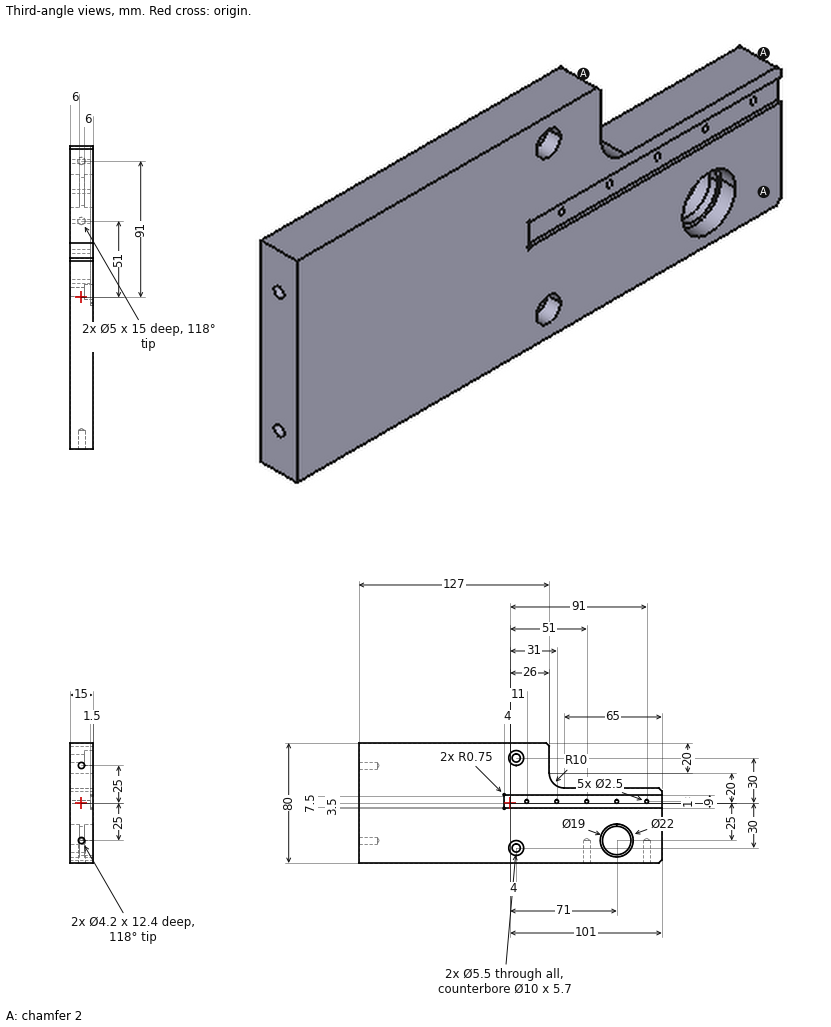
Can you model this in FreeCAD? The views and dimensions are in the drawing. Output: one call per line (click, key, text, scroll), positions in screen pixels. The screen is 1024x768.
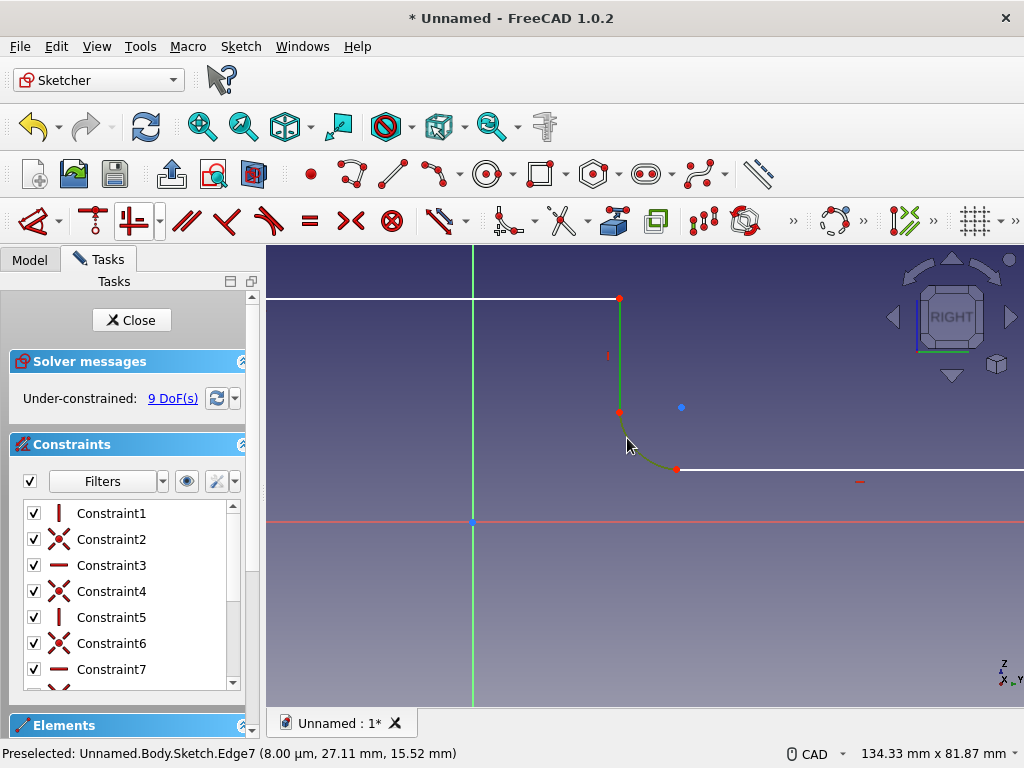
click(269, 222)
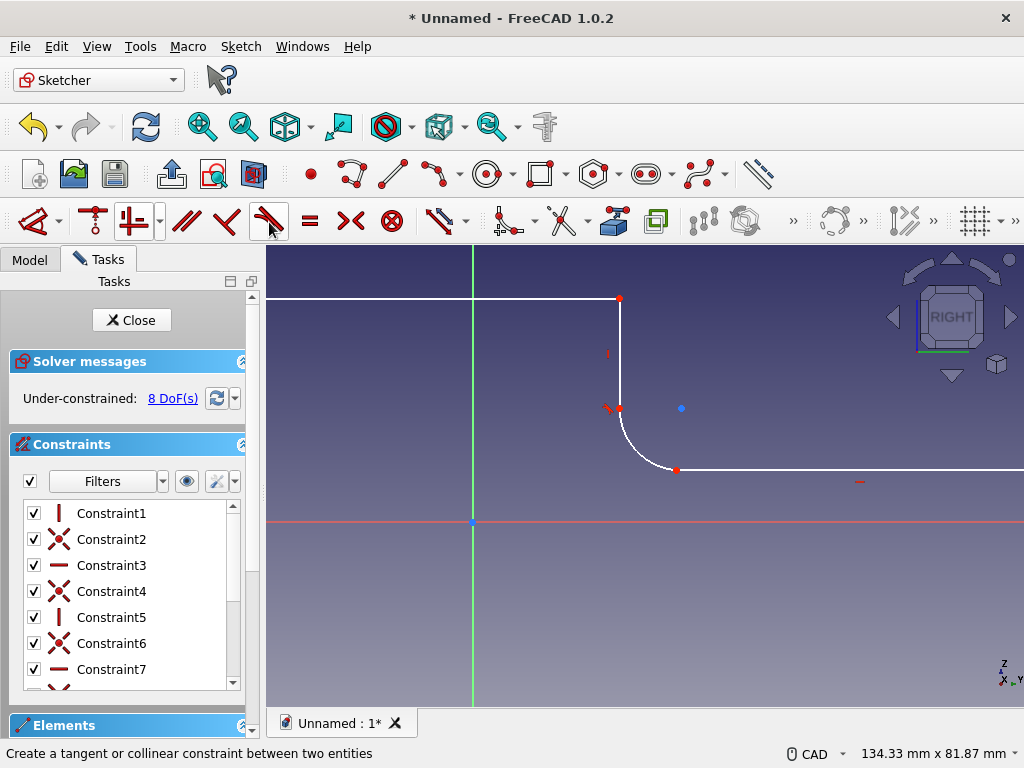
click(787, 470)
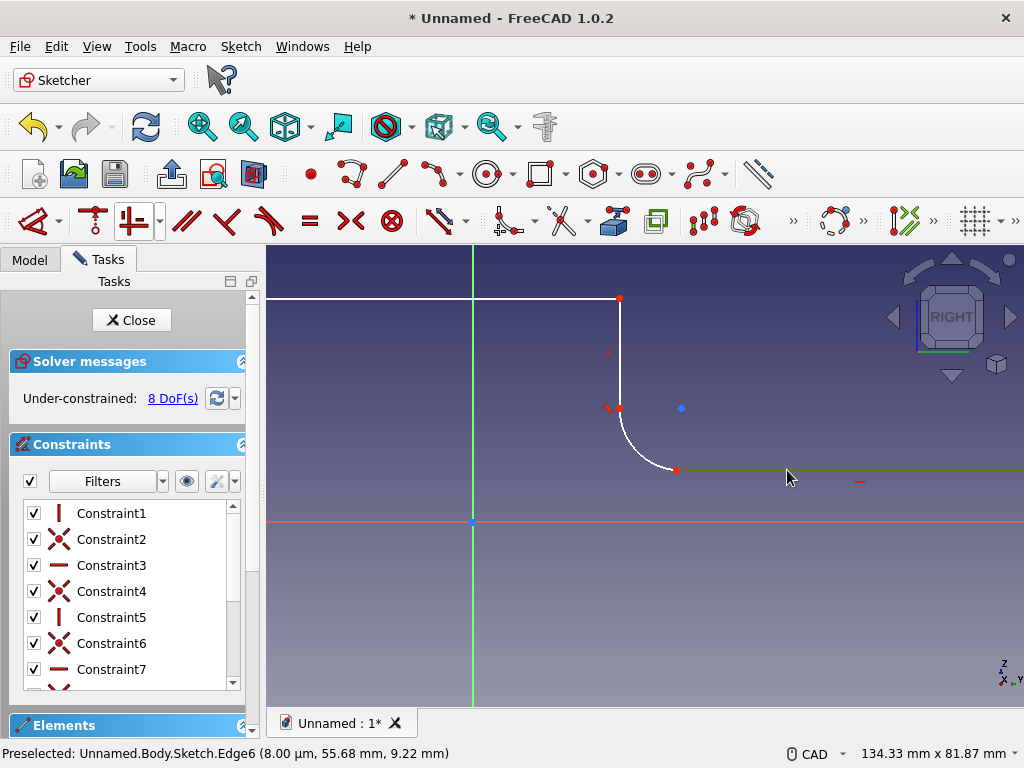
click(626, 435)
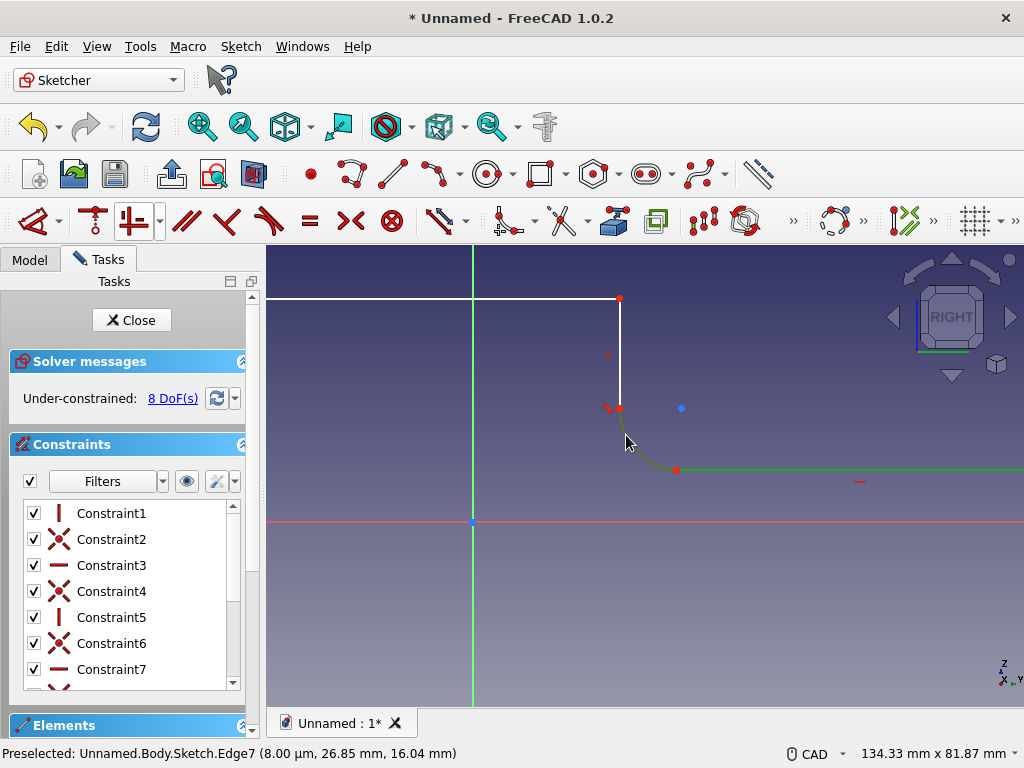
click(269, 222)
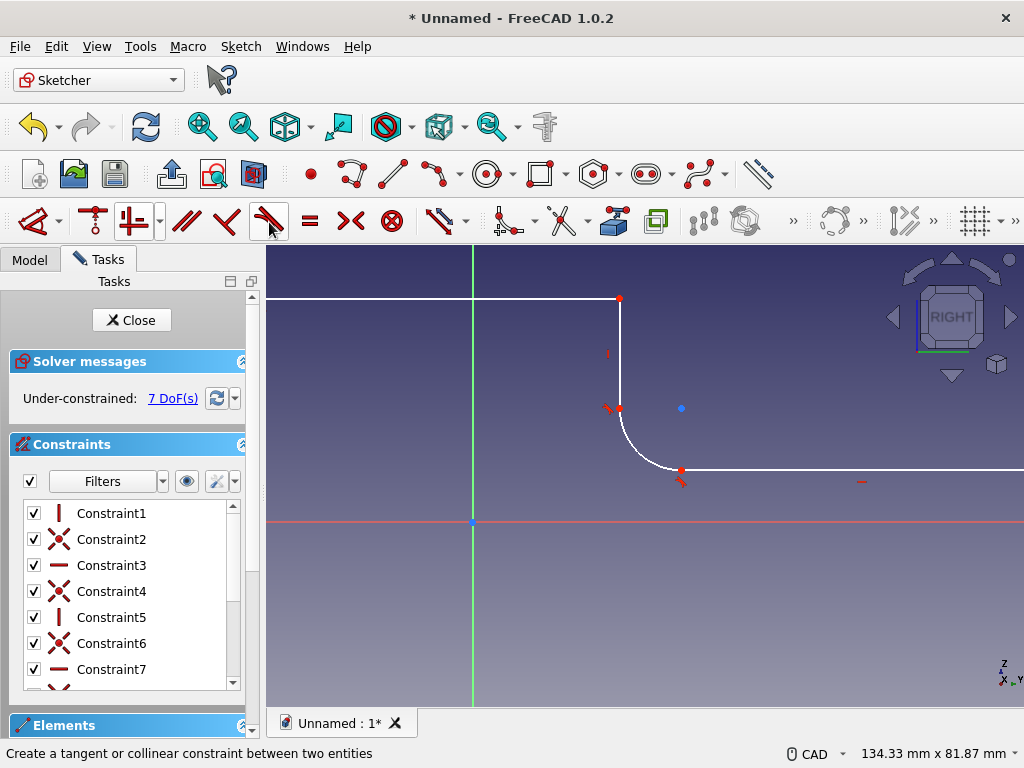
click(32, 222)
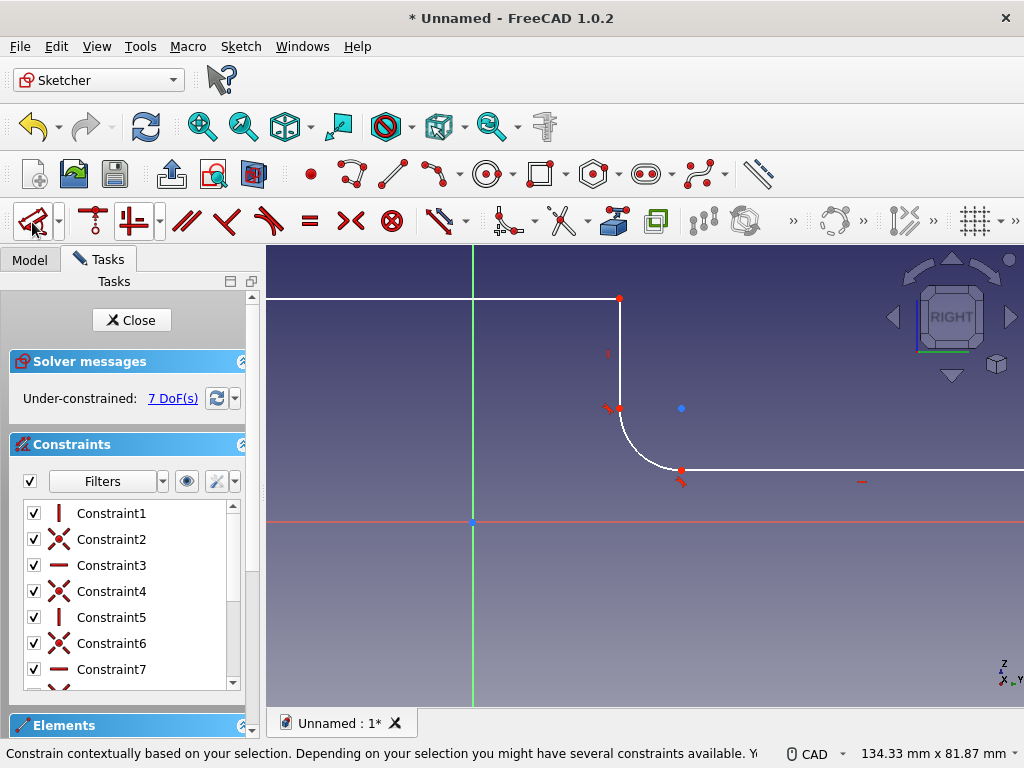
click(627, 437)
click(599, 452)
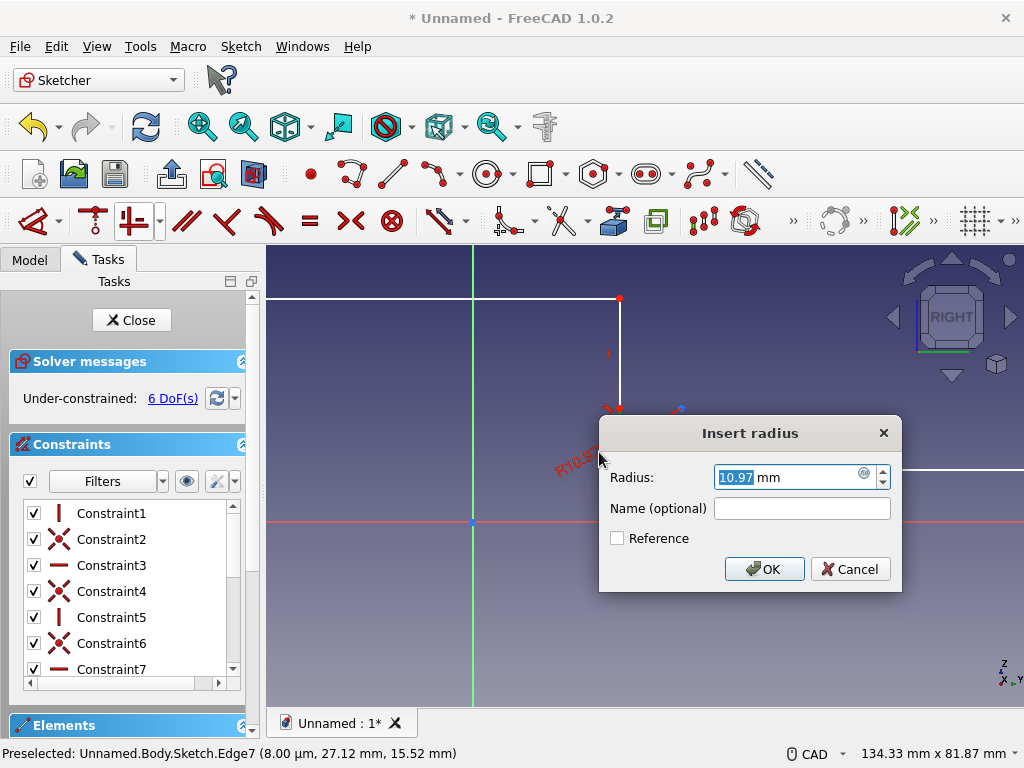
text(10)
key(Return)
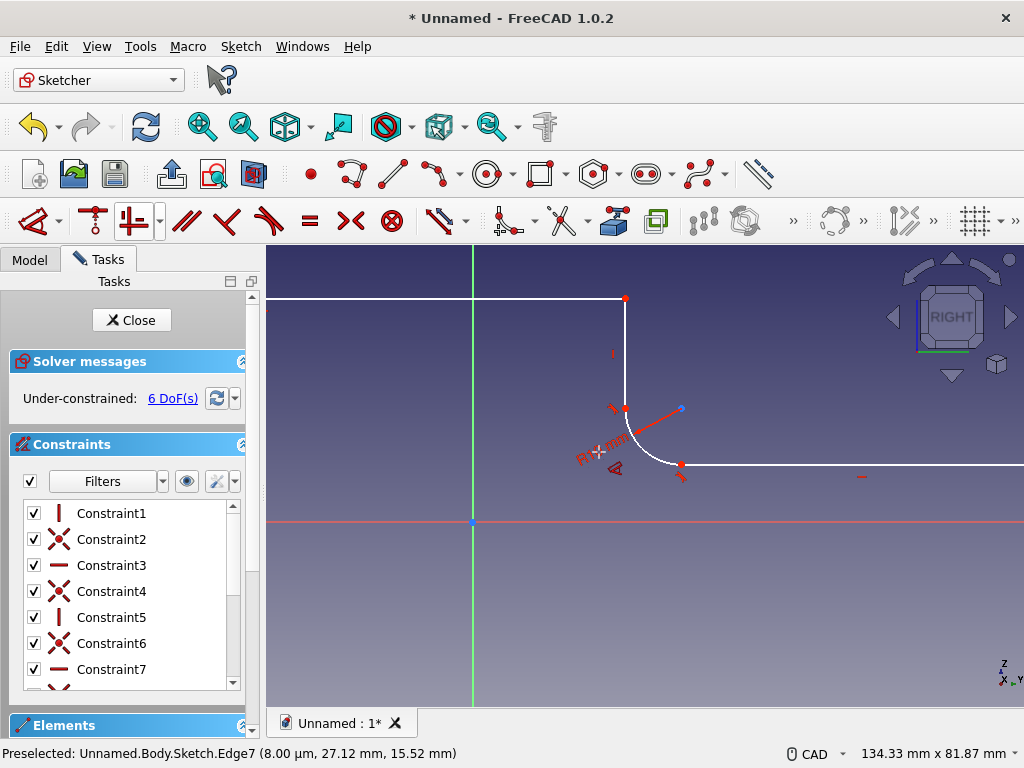
click(625, 376)
click(659, 354)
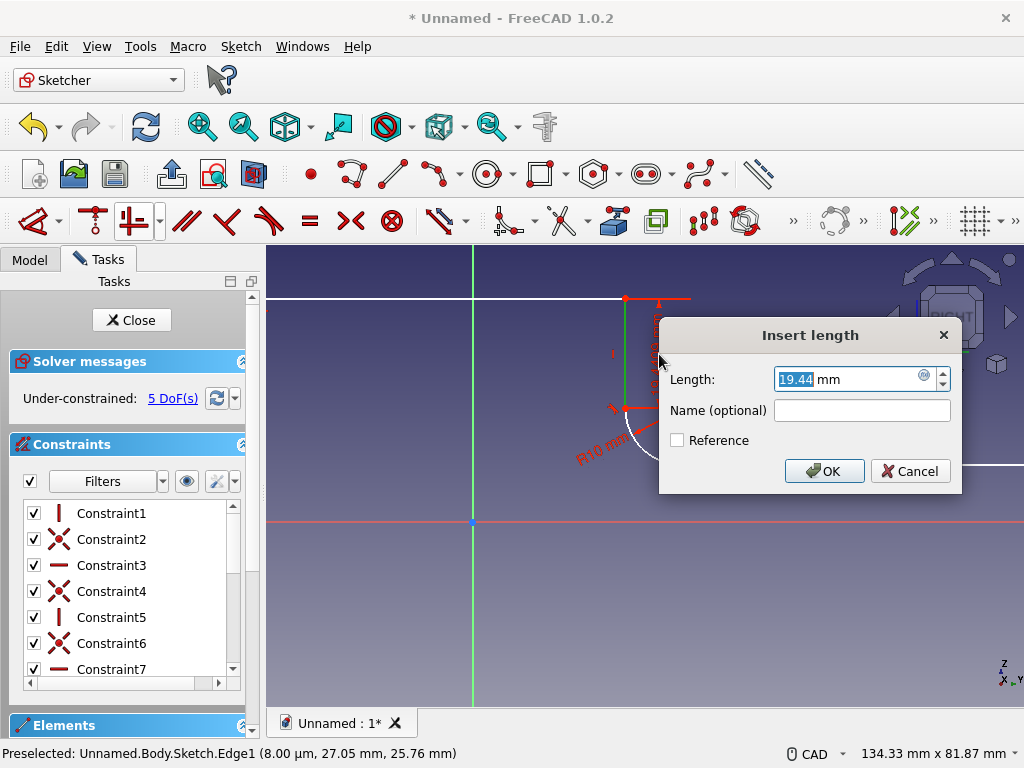
text(20)
key(Return)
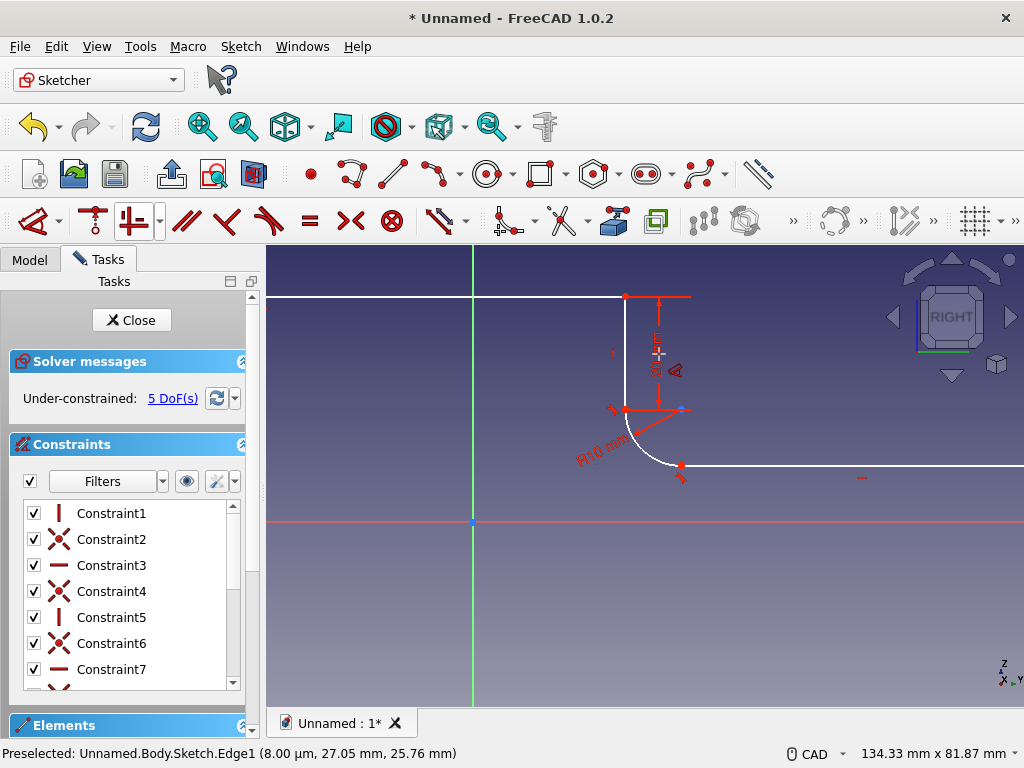
scroll(637, 449, down, 5)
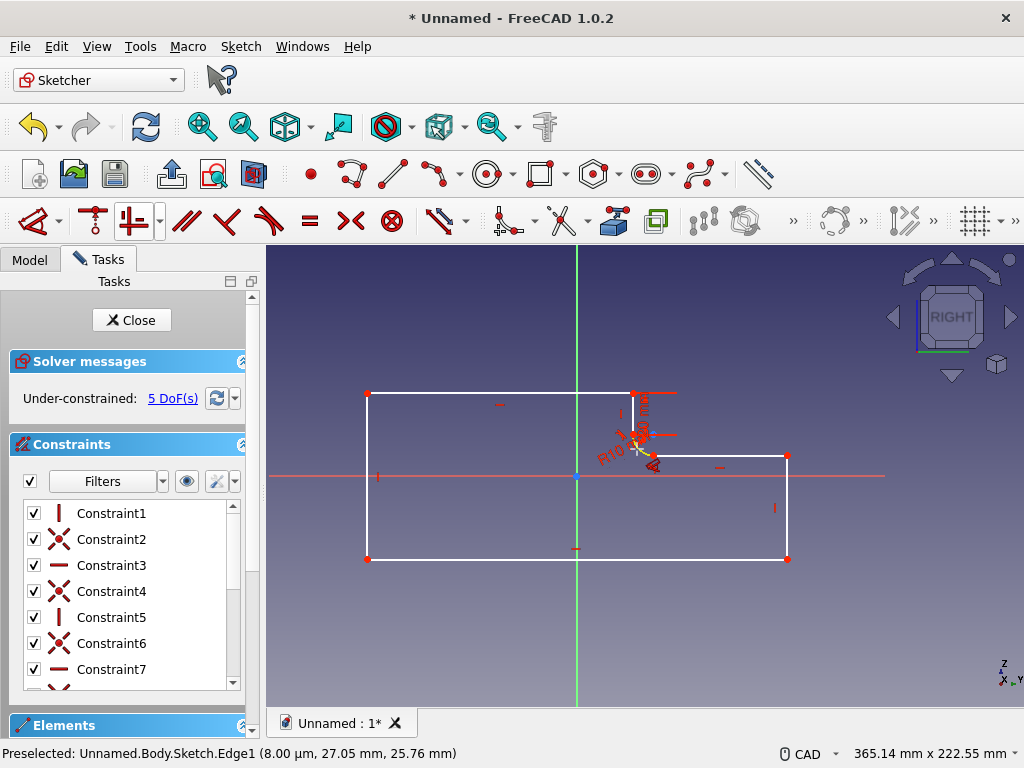
click(367, 443)
click(333, 438)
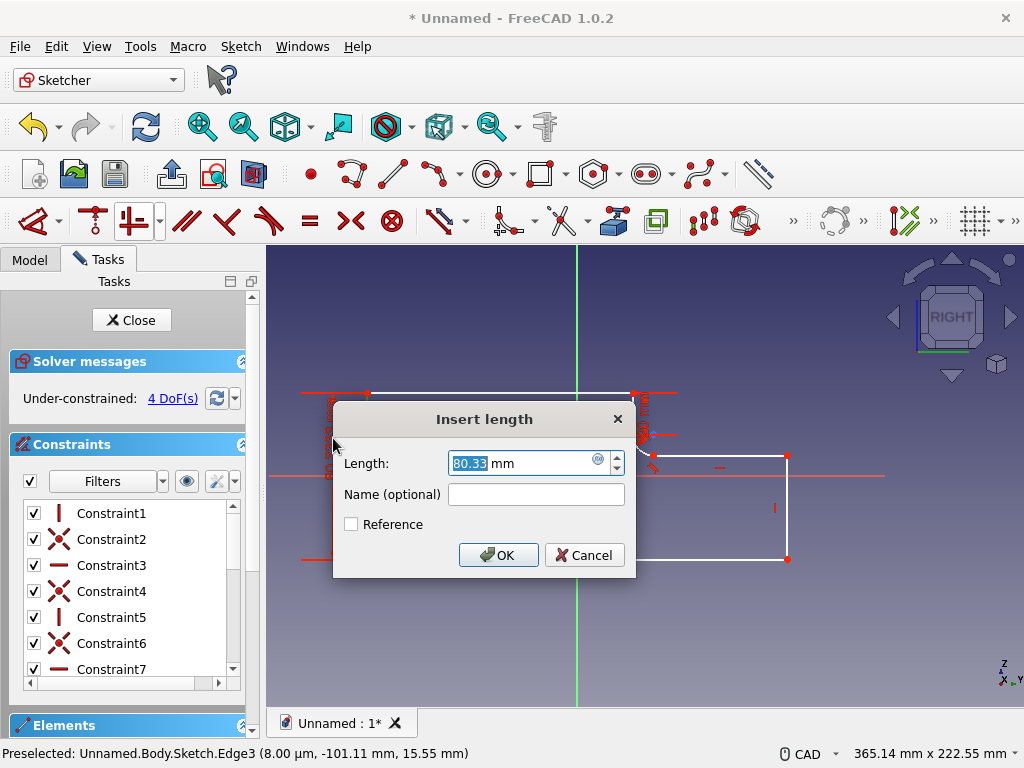
text(80)
key(Return)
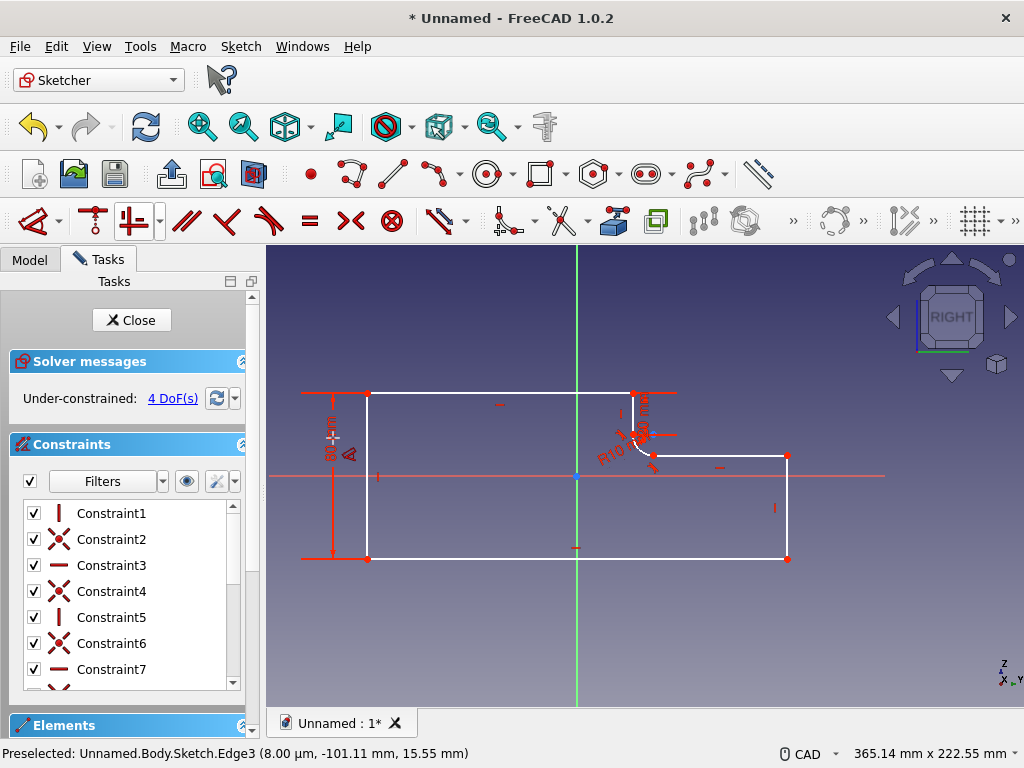
click(747, 456)
click(720, 422)